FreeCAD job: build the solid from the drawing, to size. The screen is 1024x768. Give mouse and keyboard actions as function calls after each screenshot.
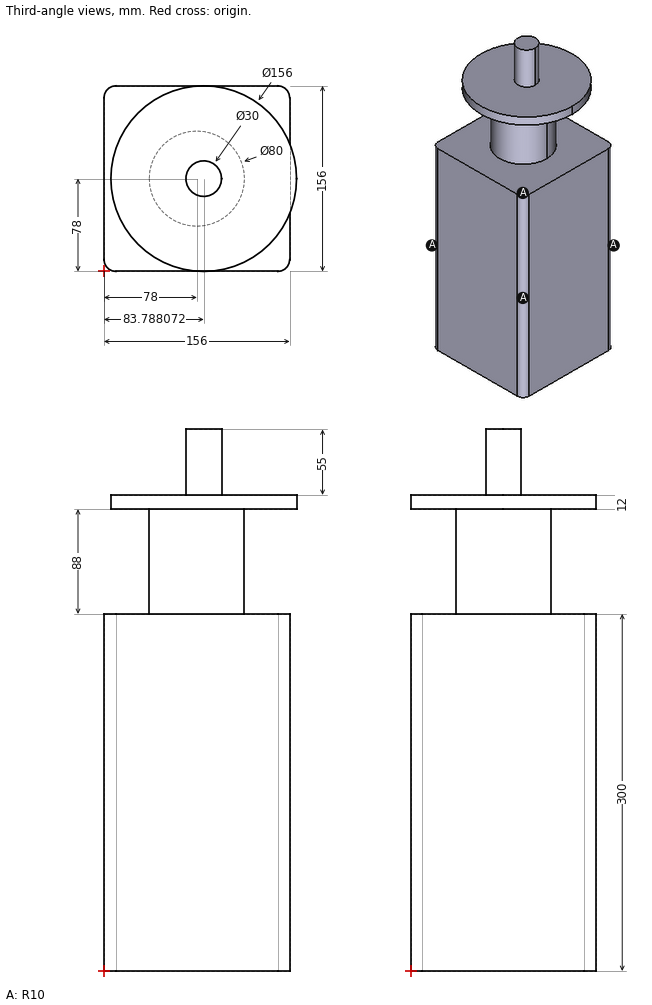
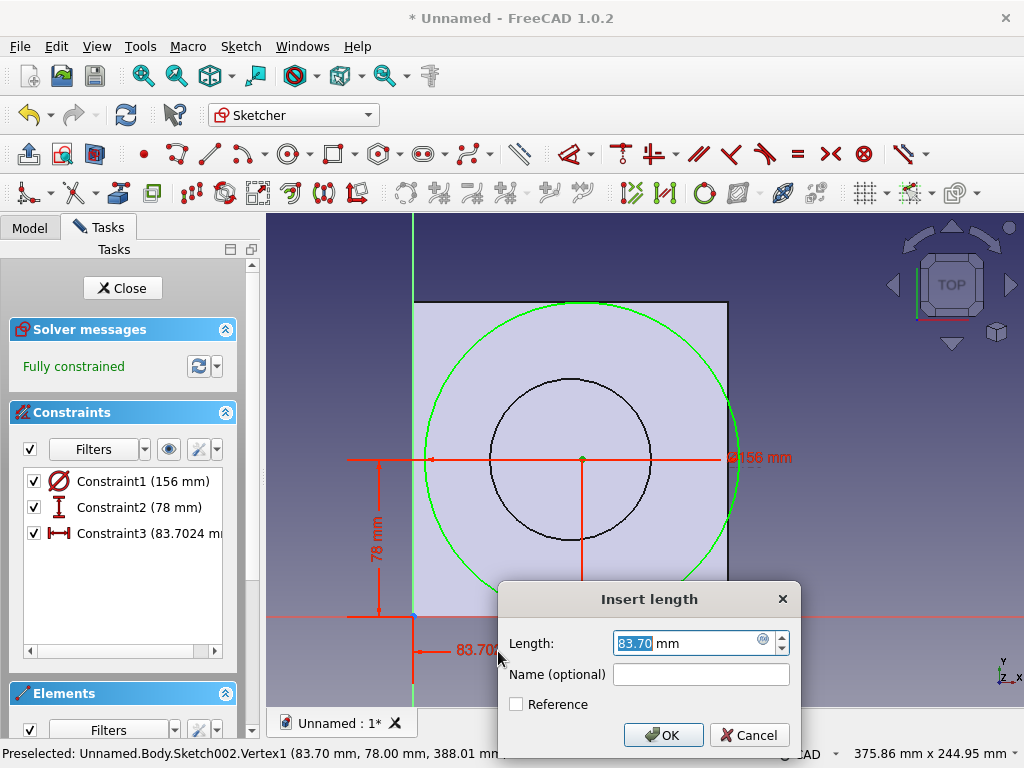
text(83.788072)
key(Return)
key(Escape)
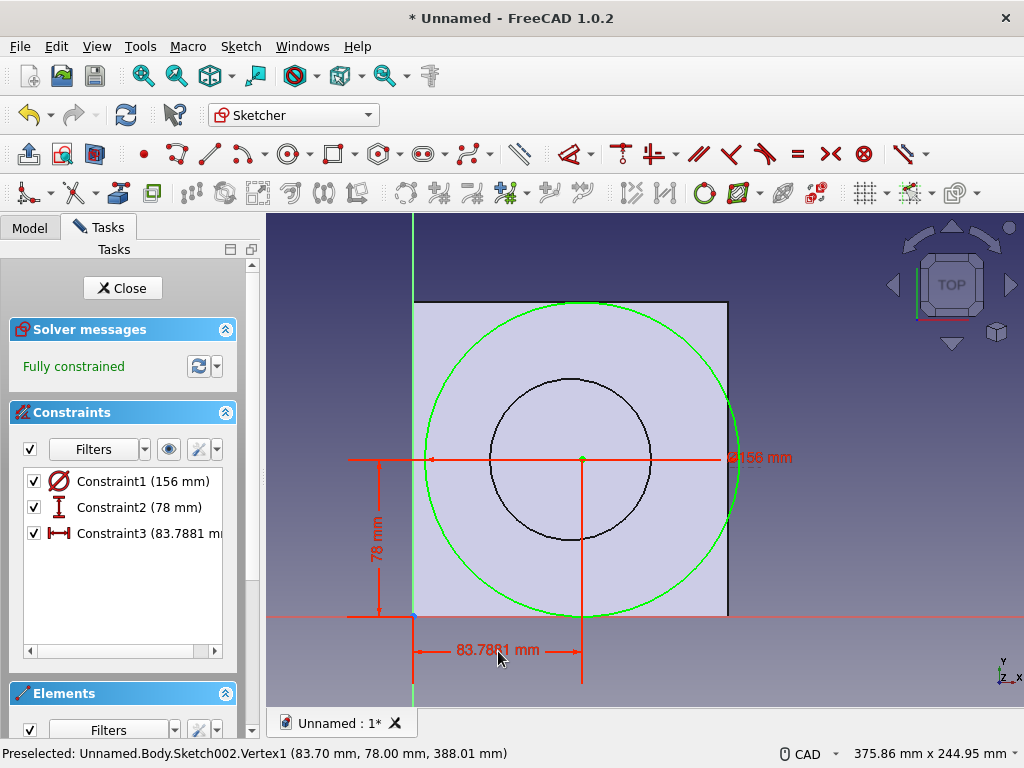
click(123, 288)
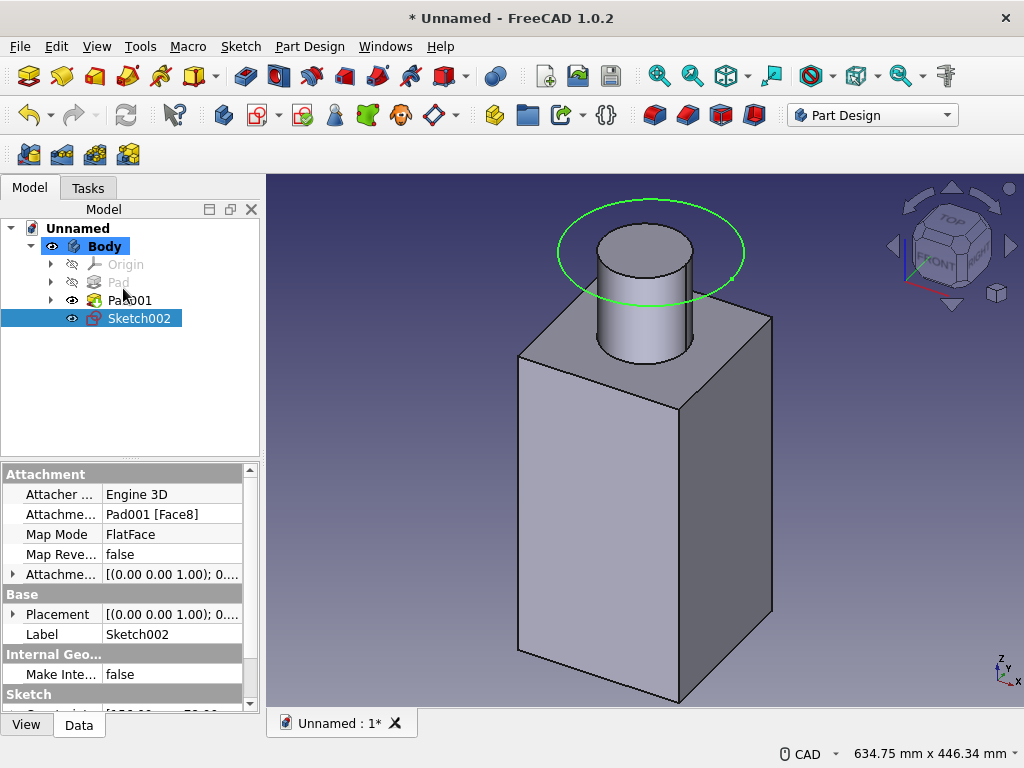
click(29, 76)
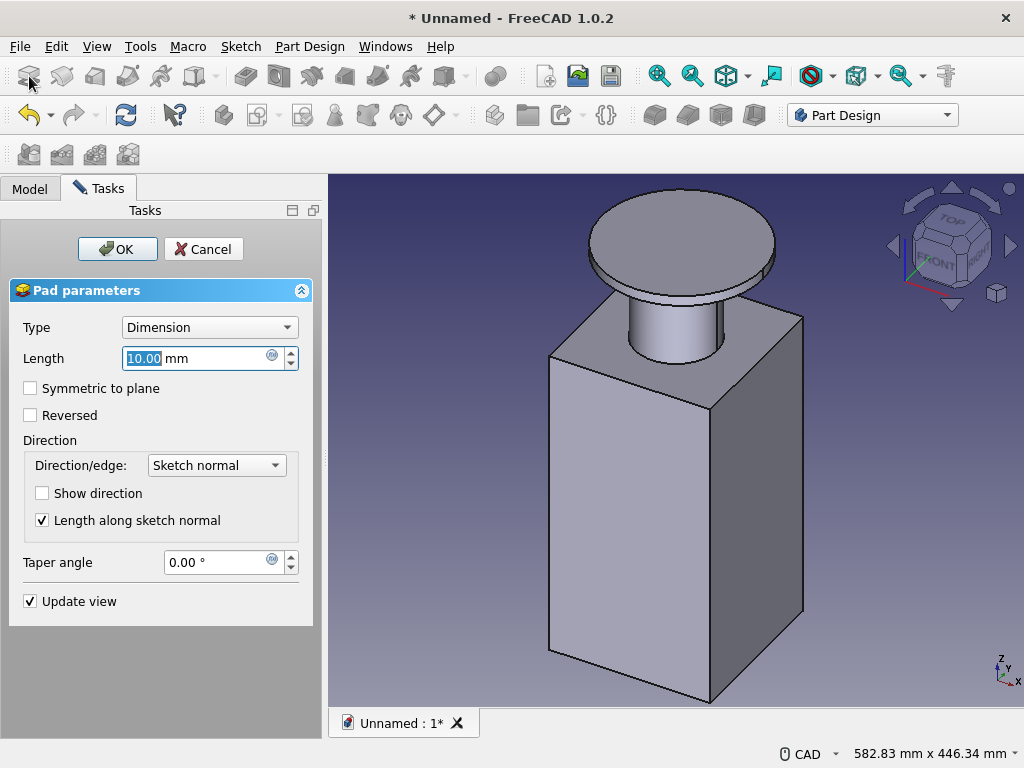
text(12)
key(Tab)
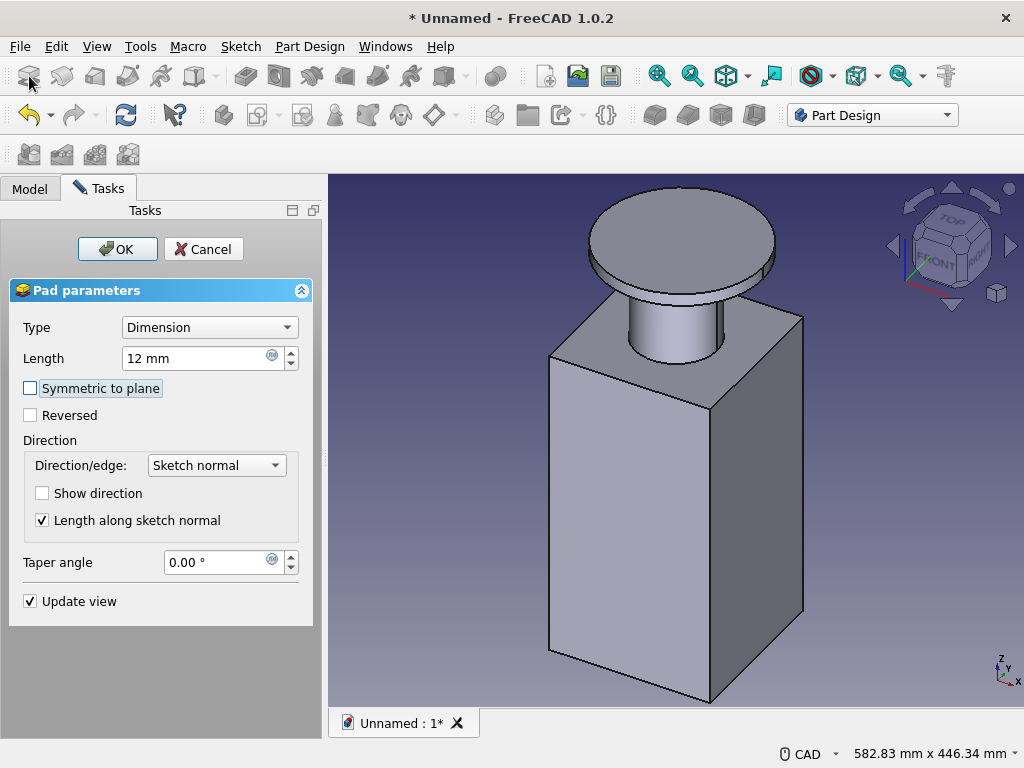
click(118, 249)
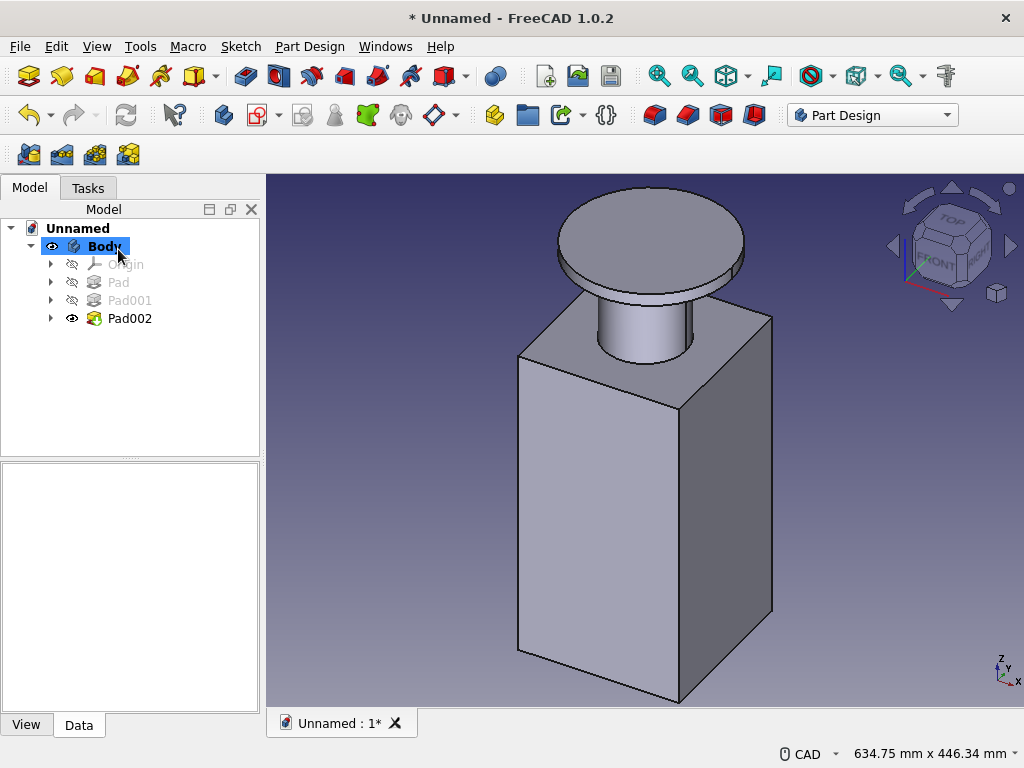
click(660, 76)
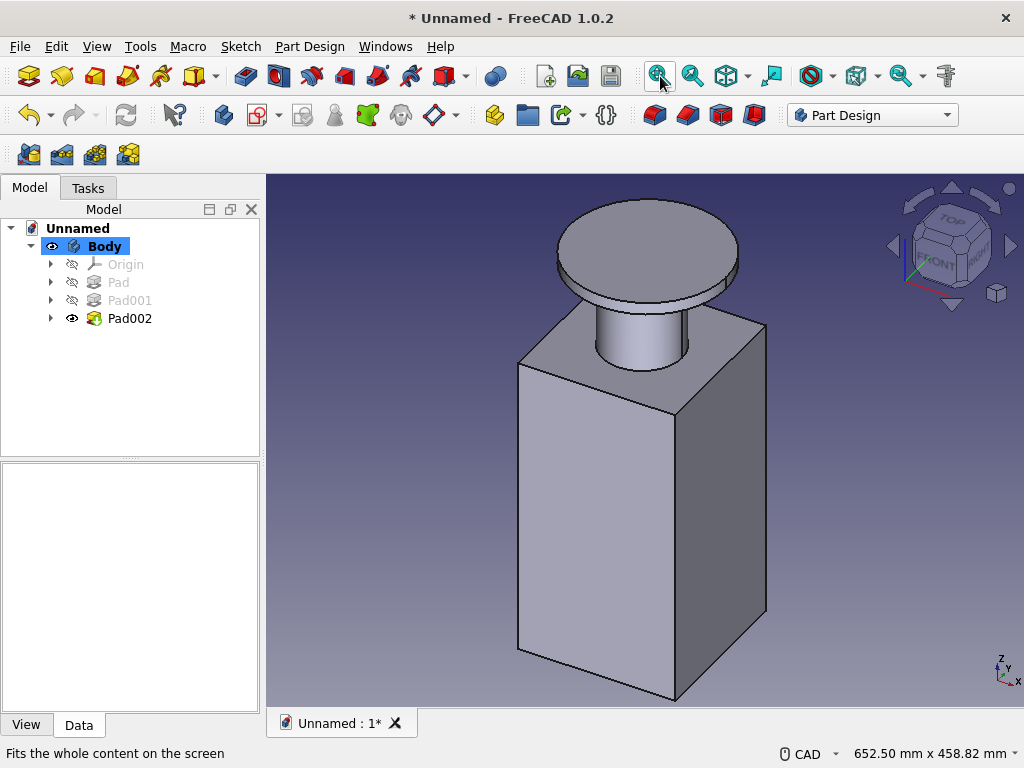
click(675, 557)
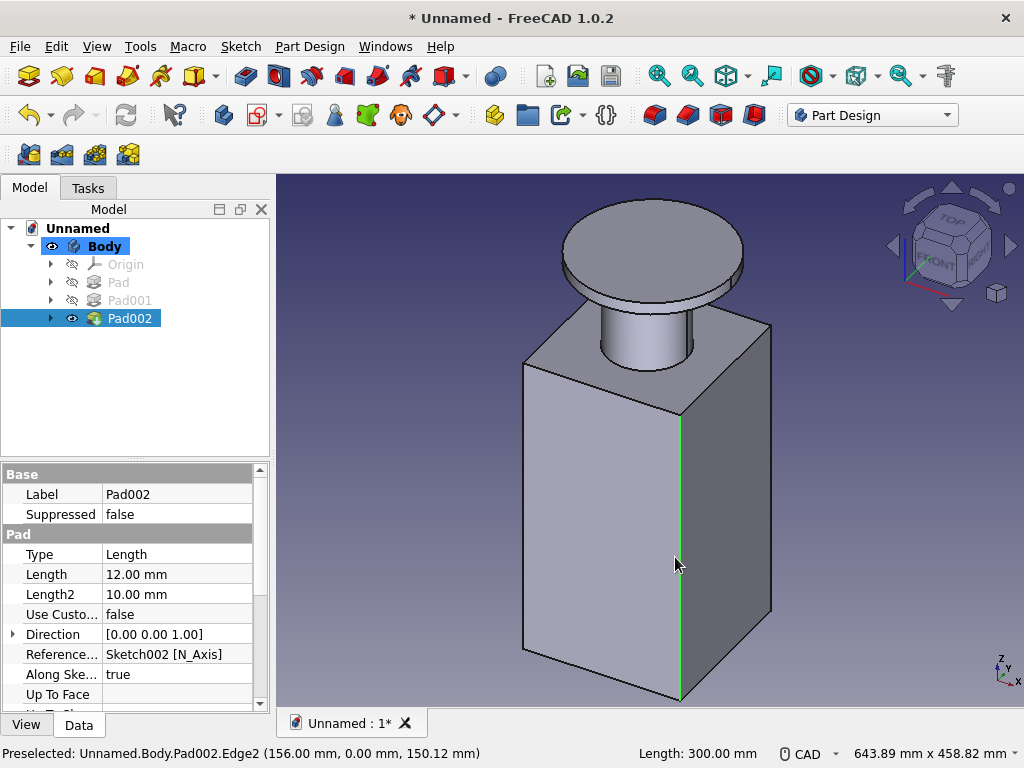
key(0)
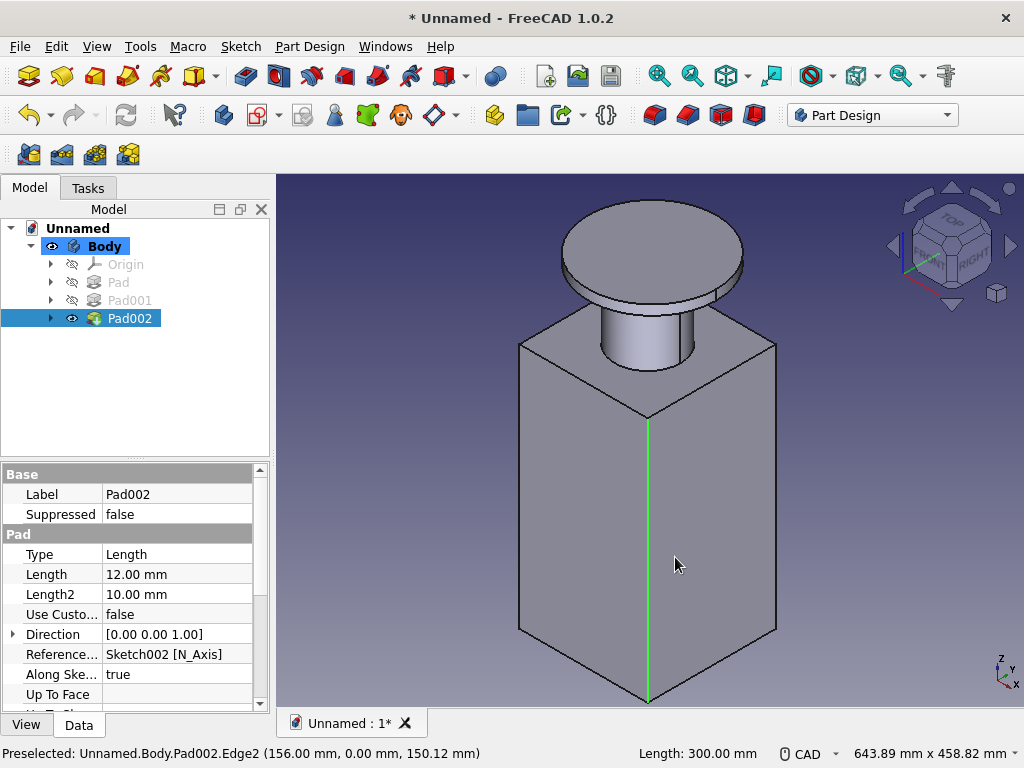
key(2)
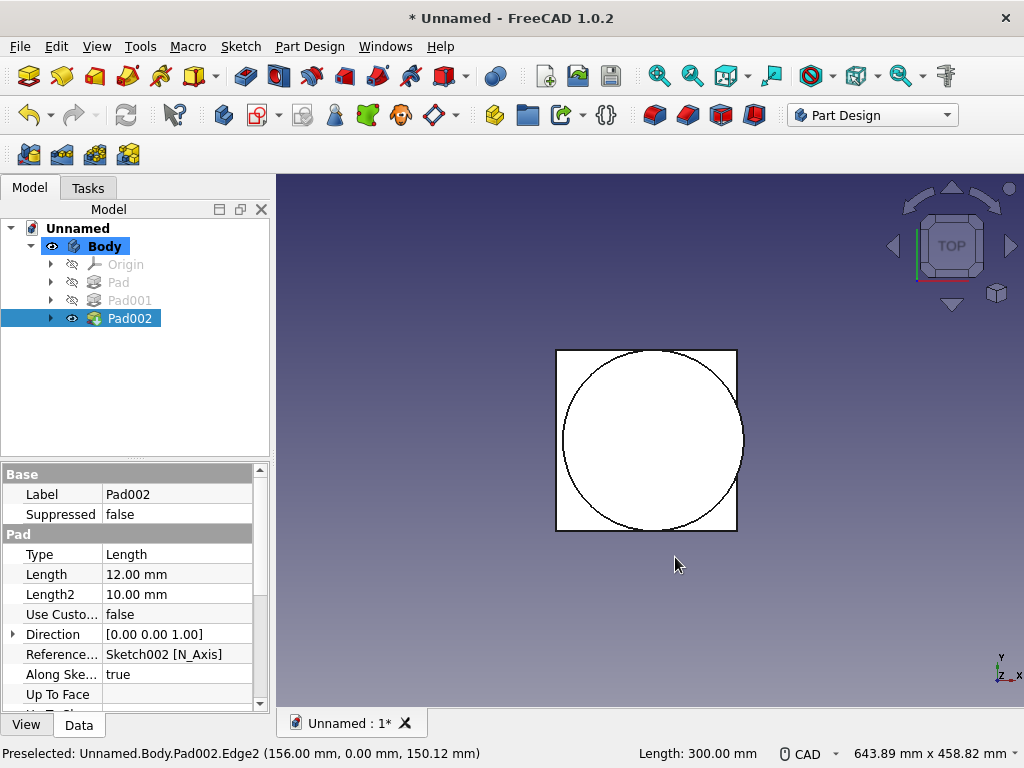
click(660, 76)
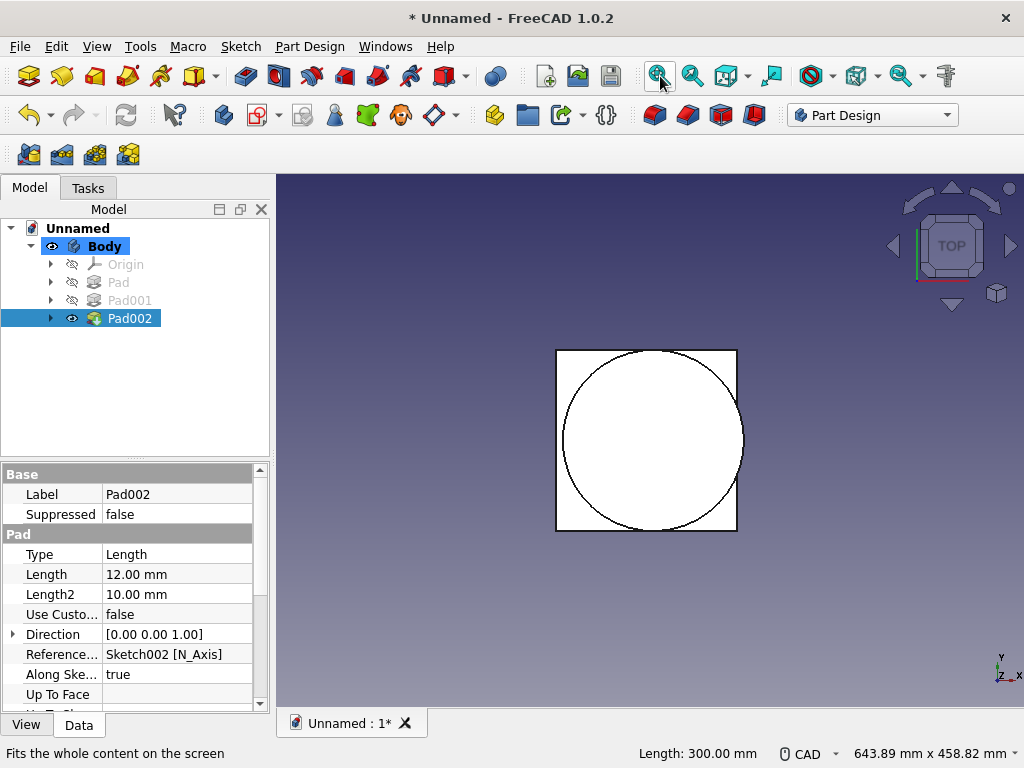
key(1)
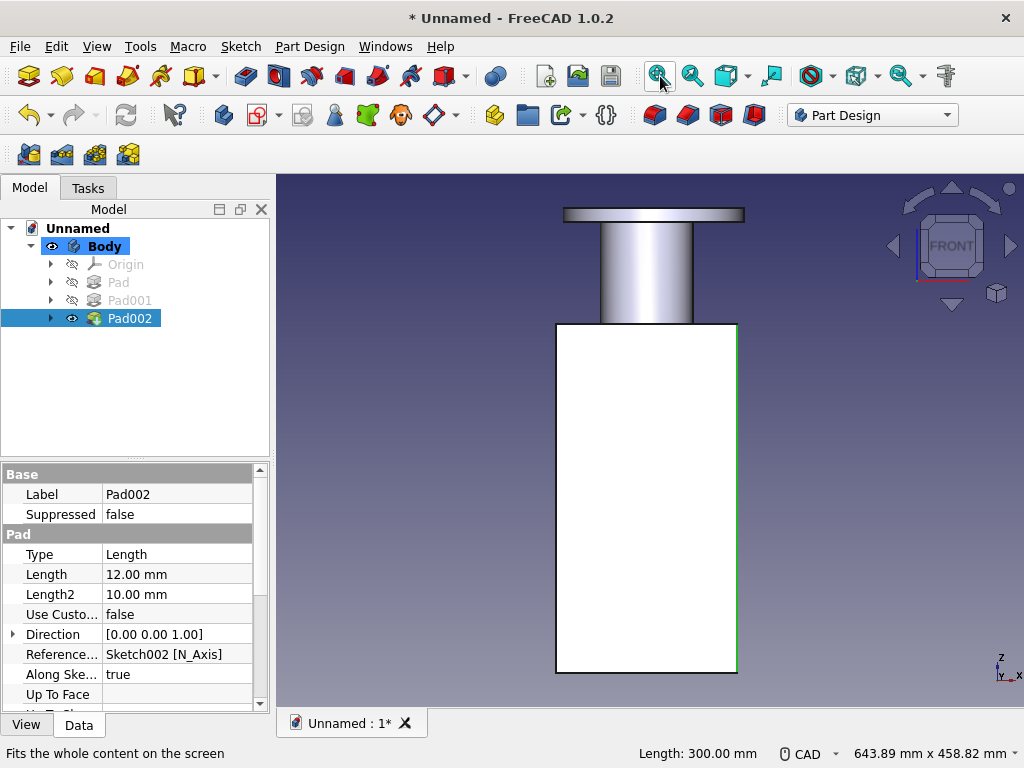
click(556, 498, ctrl)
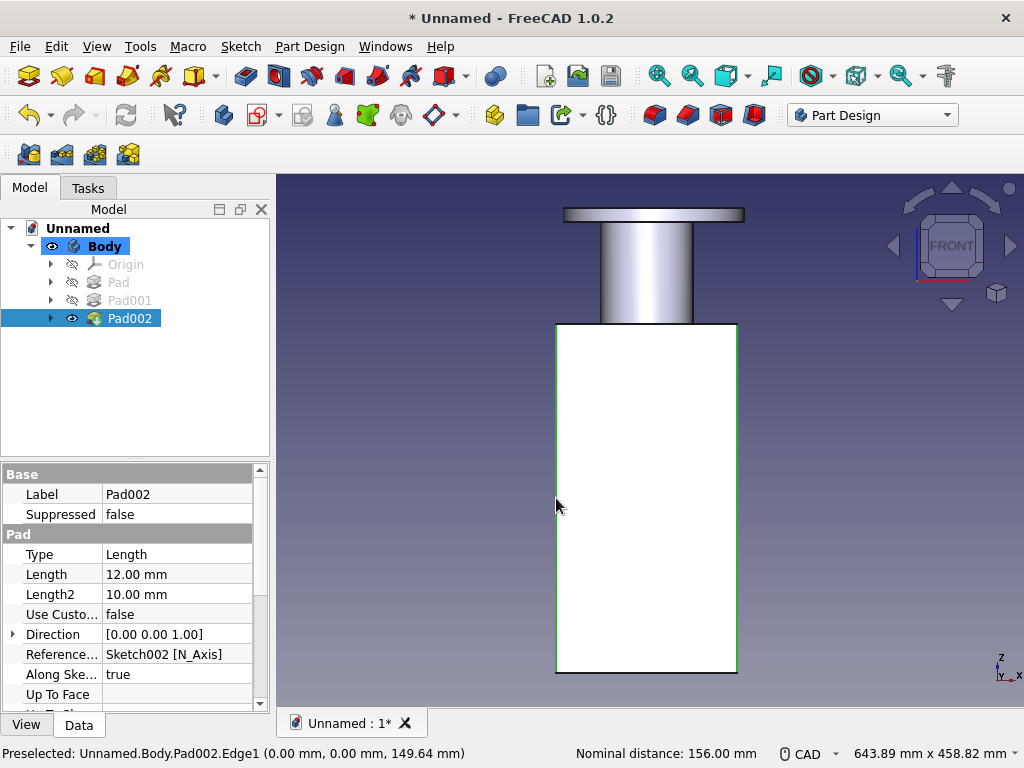
key(3)